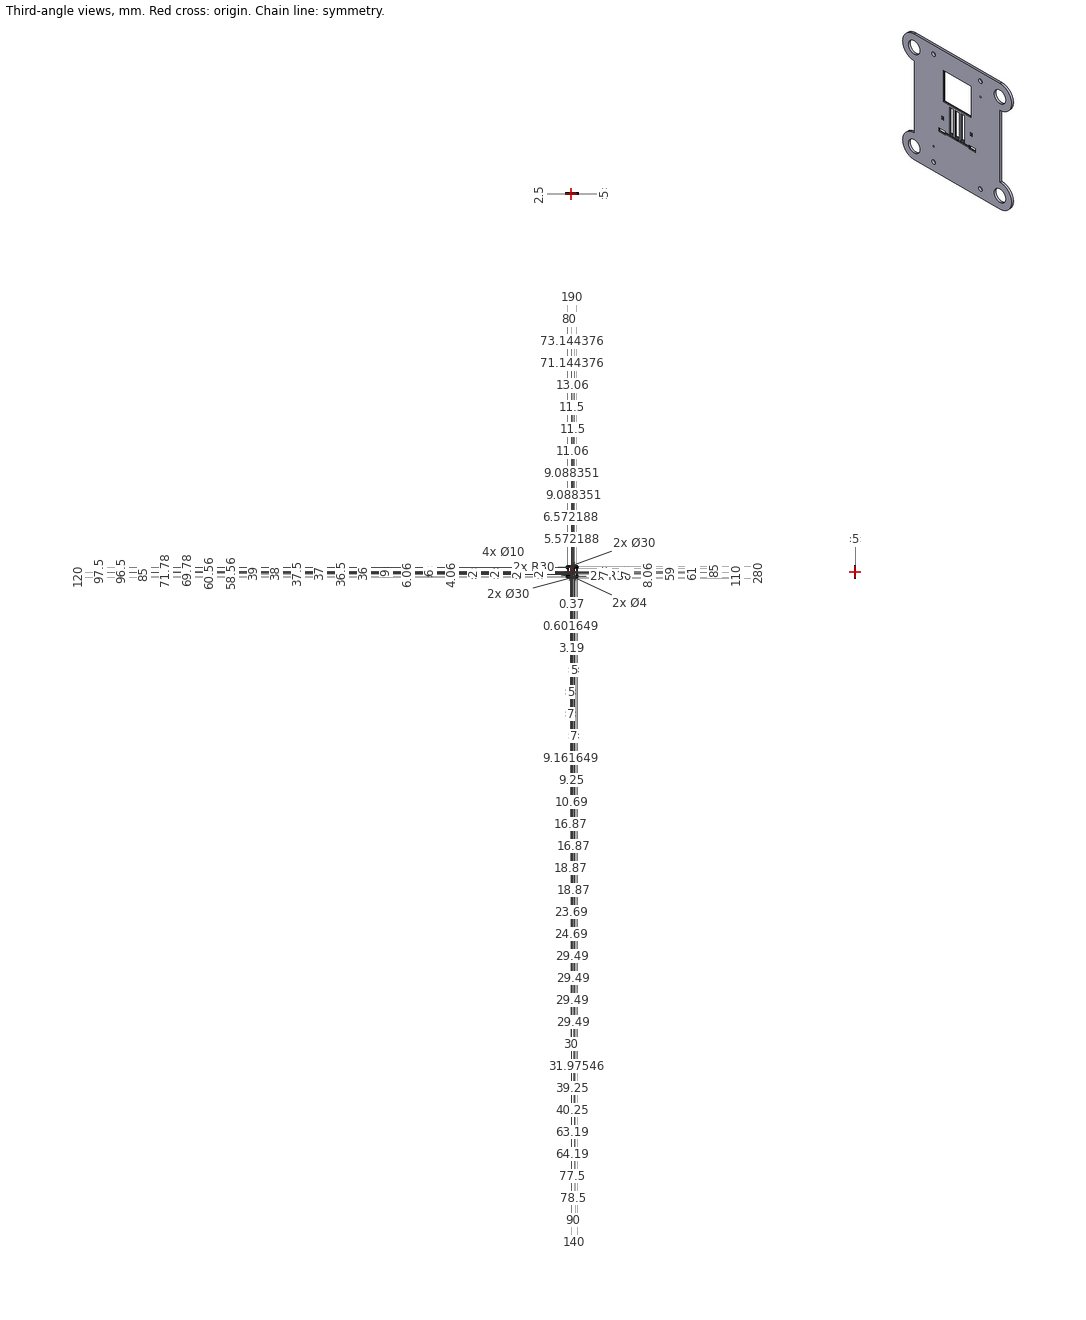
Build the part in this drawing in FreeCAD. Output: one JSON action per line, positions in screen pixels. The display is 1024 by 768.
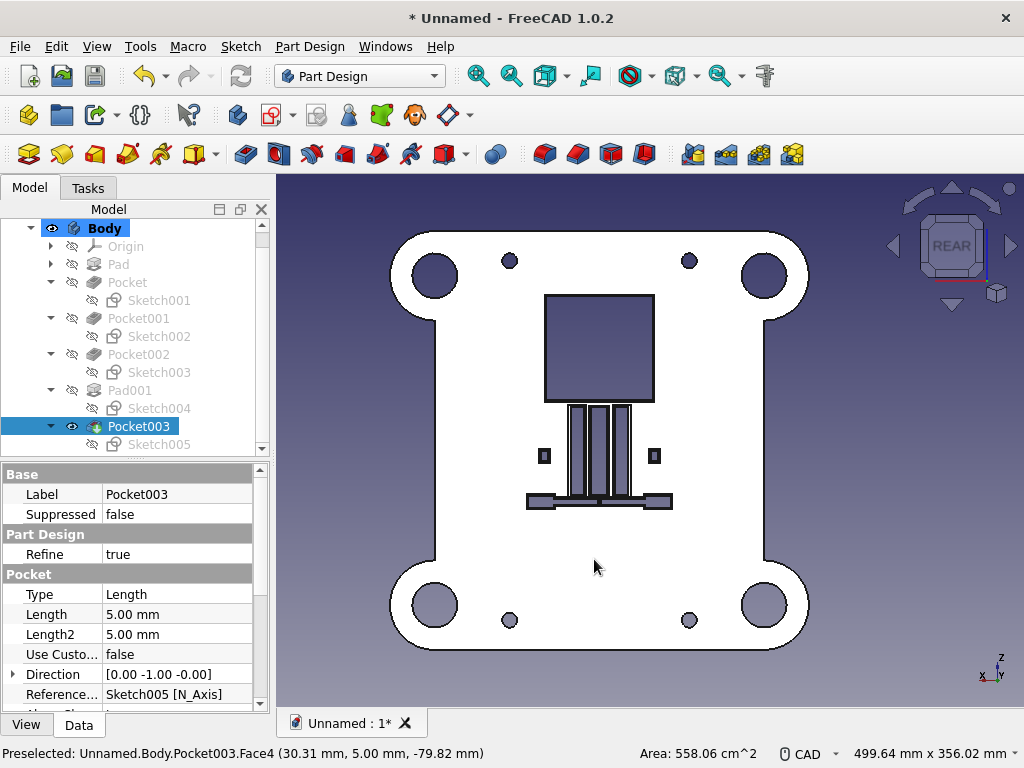
{"action": "left_click", "coordinate": [270, 116]}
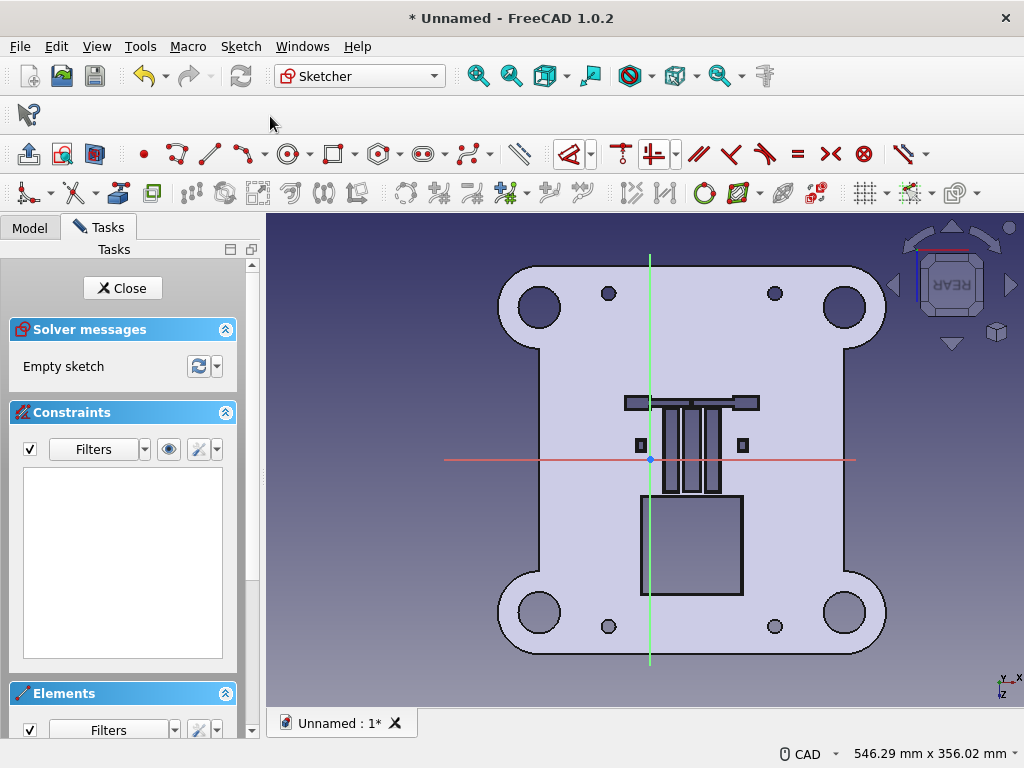
{"action": "left_click", "coordinate": [288, 154]}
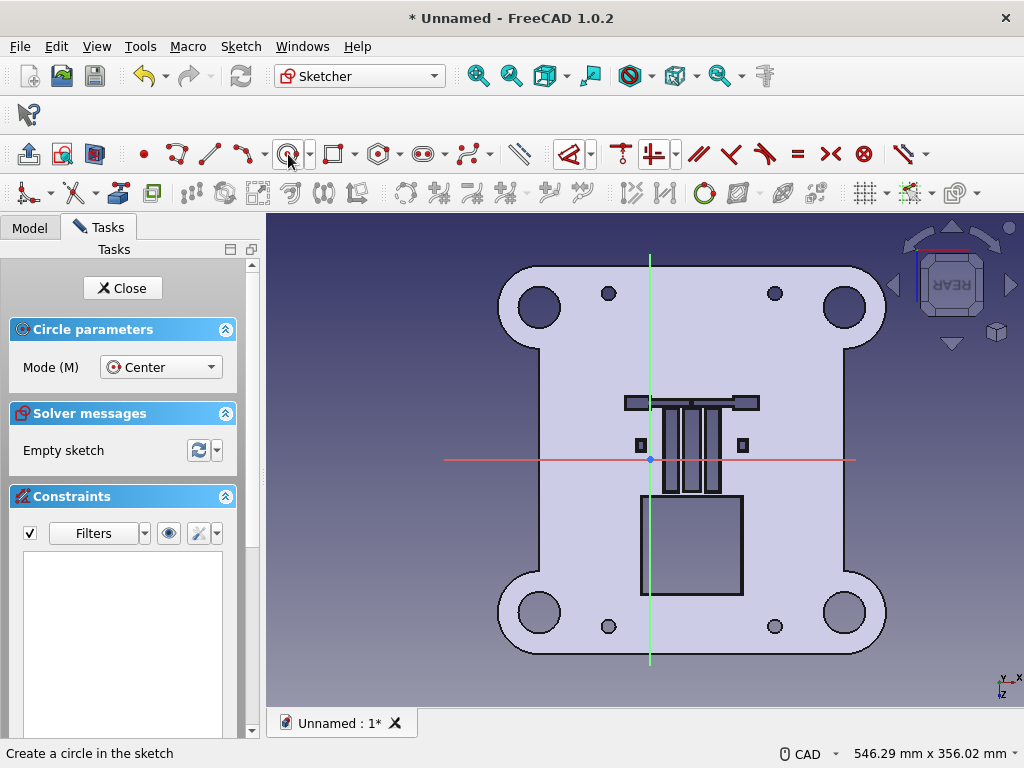
{"action": "scroll", "coordinate": [609, 342], "scroll_direction": "up", "scroll_amount": 11}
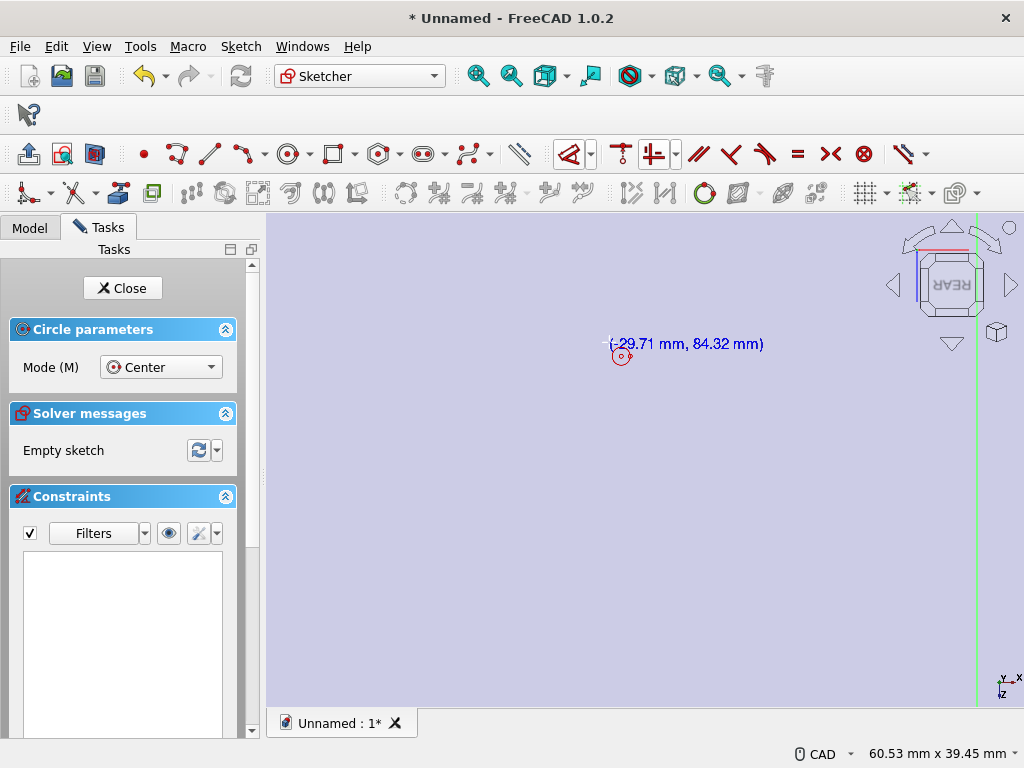
{"action": "scroll", "coordinate": [455, 312], "scroll_direction": "down", "scroll_amount": 10}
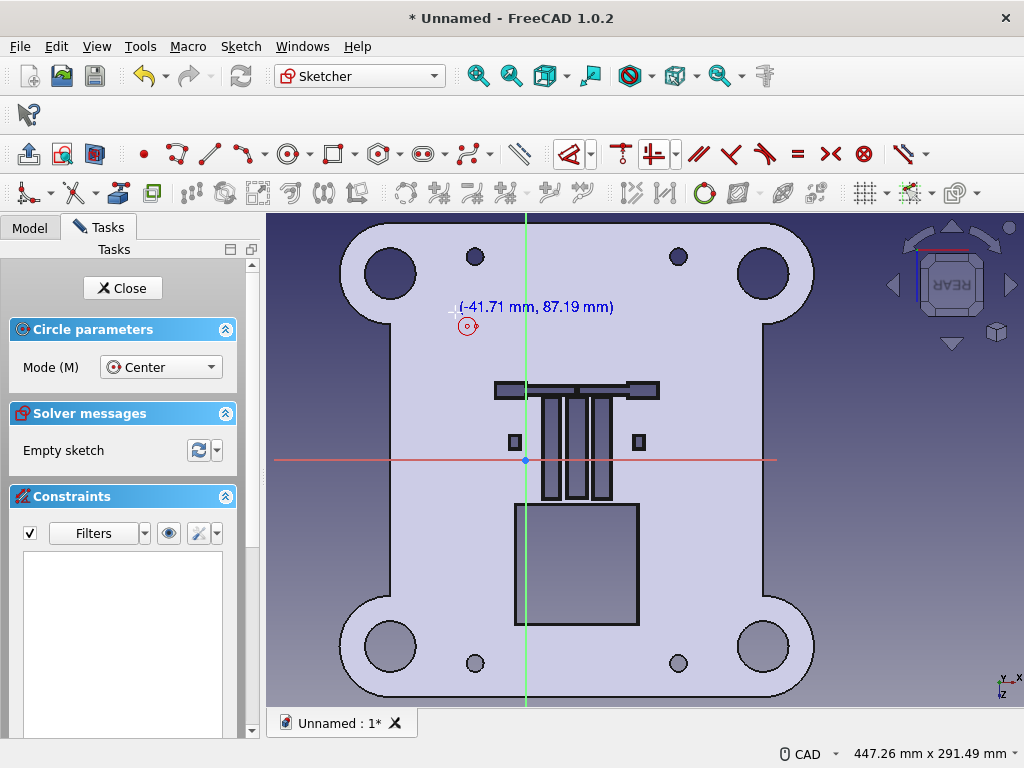
{"action": "left_click", "coordinate": [475, 316]}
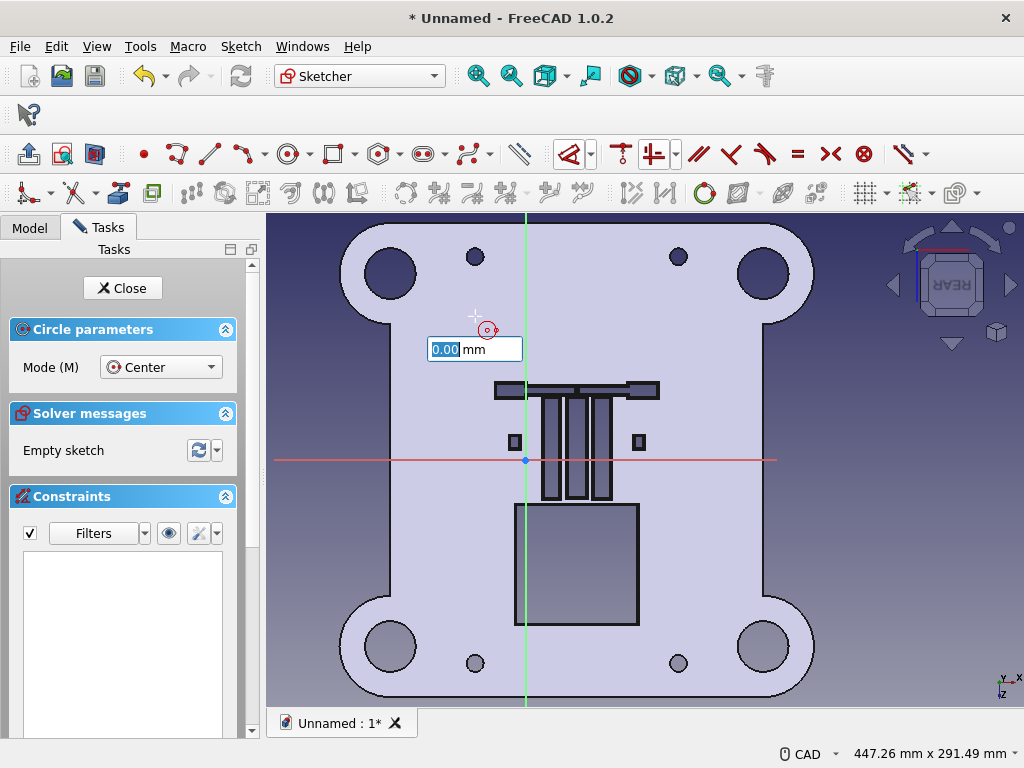
{"action": "scroll", "coordinate": [477, 314], "scroll_direction": "up", "scroll_amount": 8}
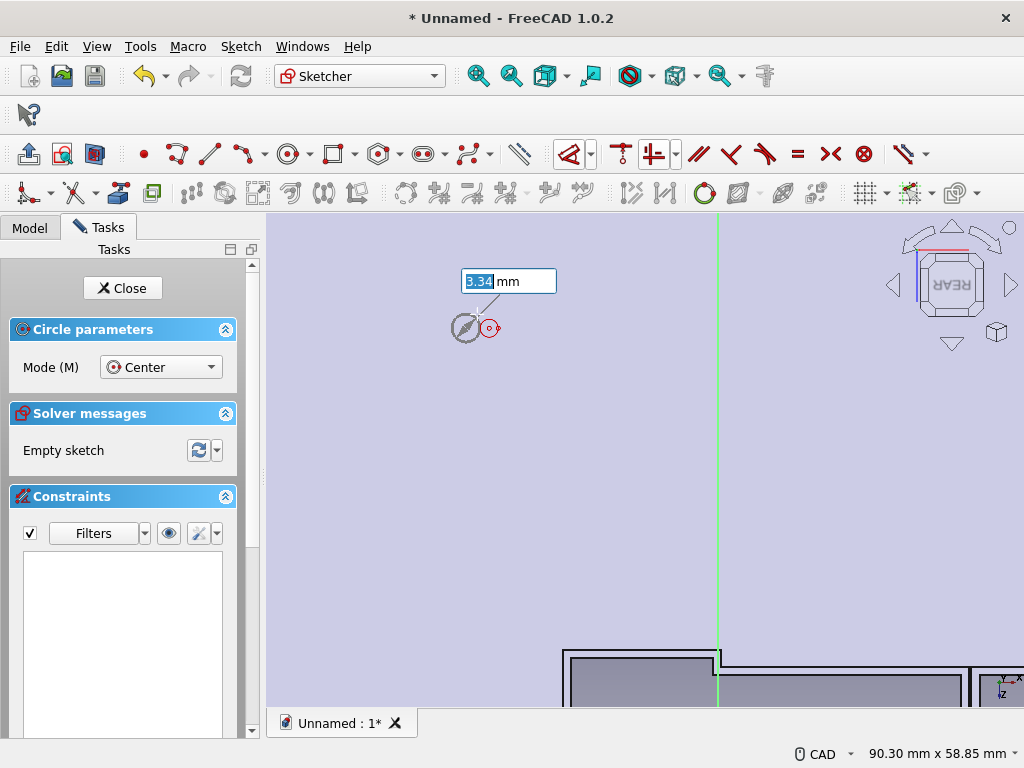
{"action": "left_click", "coordinate": [478, 311]}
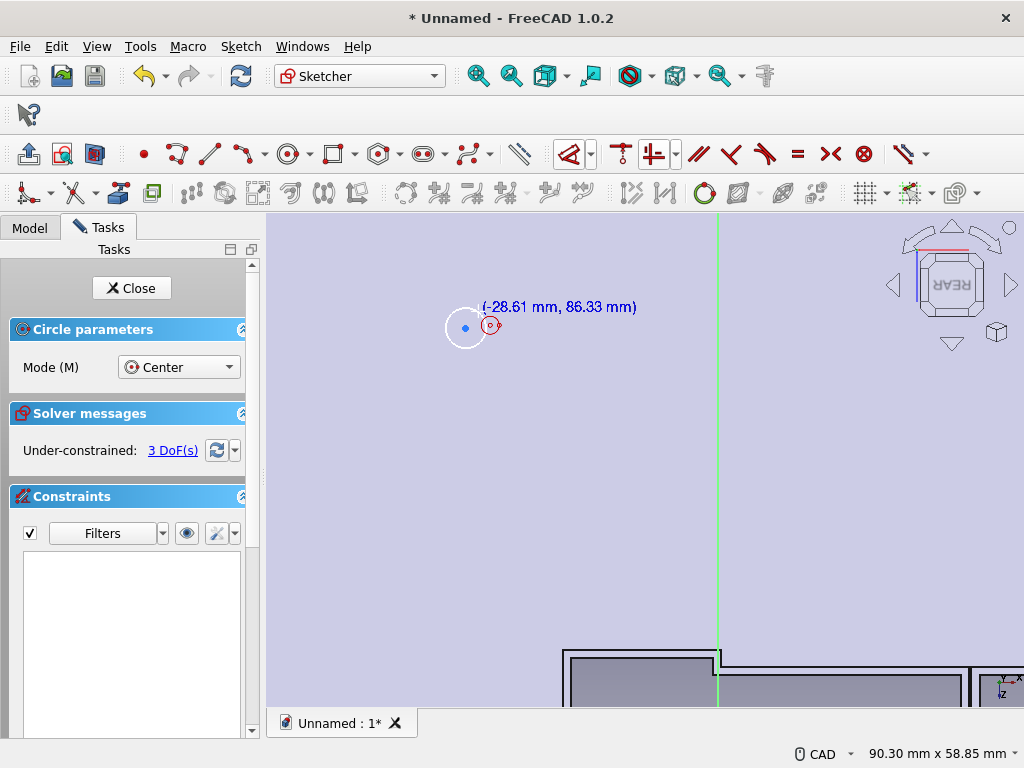
{"action": "scroll", "coordinate": [477, 314], "scroll_direction": "down", "scroll_amount": 8}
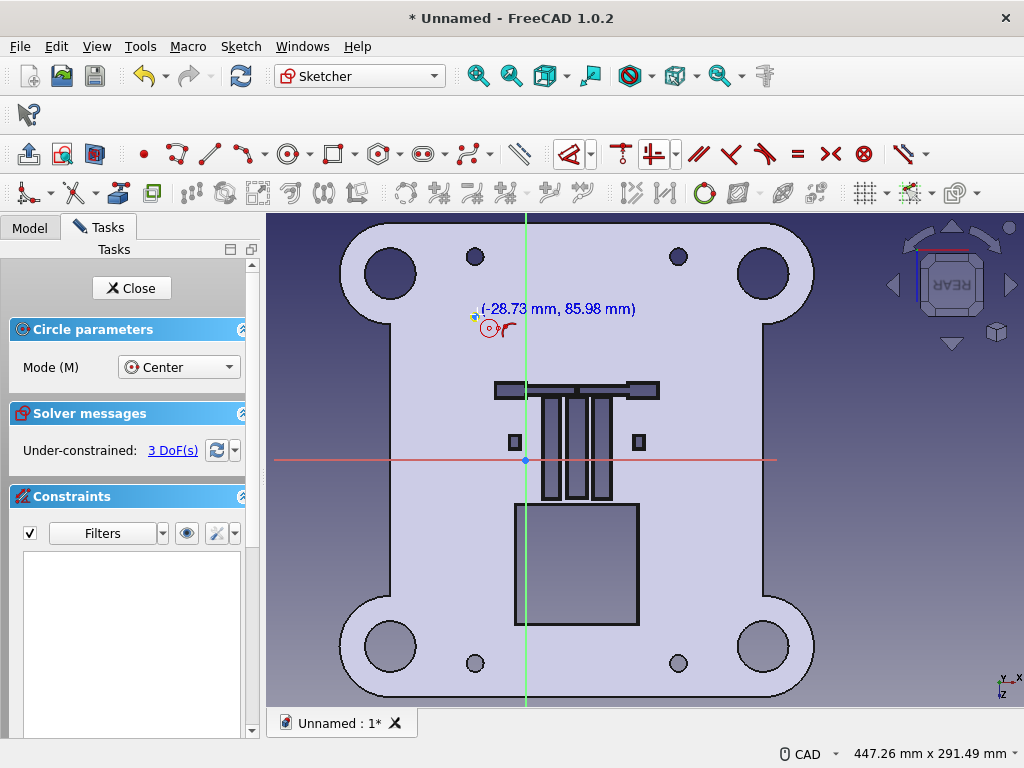
{"action": "scroll", "coordinate": [678, 604], "scroll_direction": "up", "scroll_amount": 10}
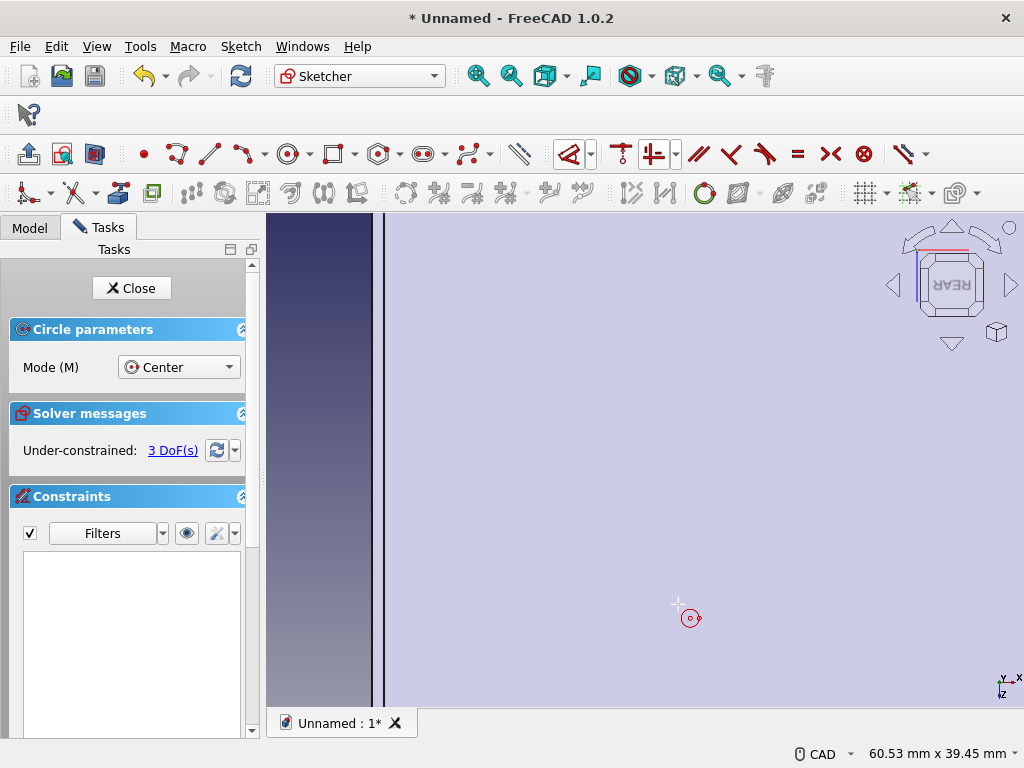
{"action": "scroll", "coordinate": [678, 605], "scroll_direction": "down", "scroll_amount": 10}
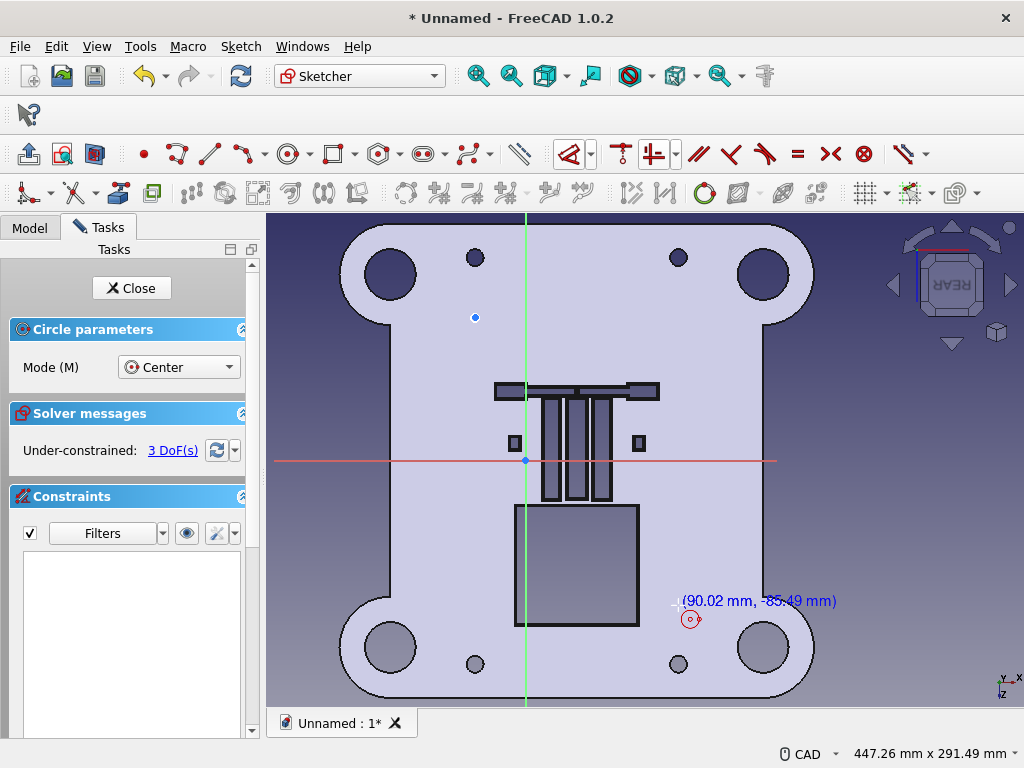
{"action": "left_click", "coordinate": [678, 605]}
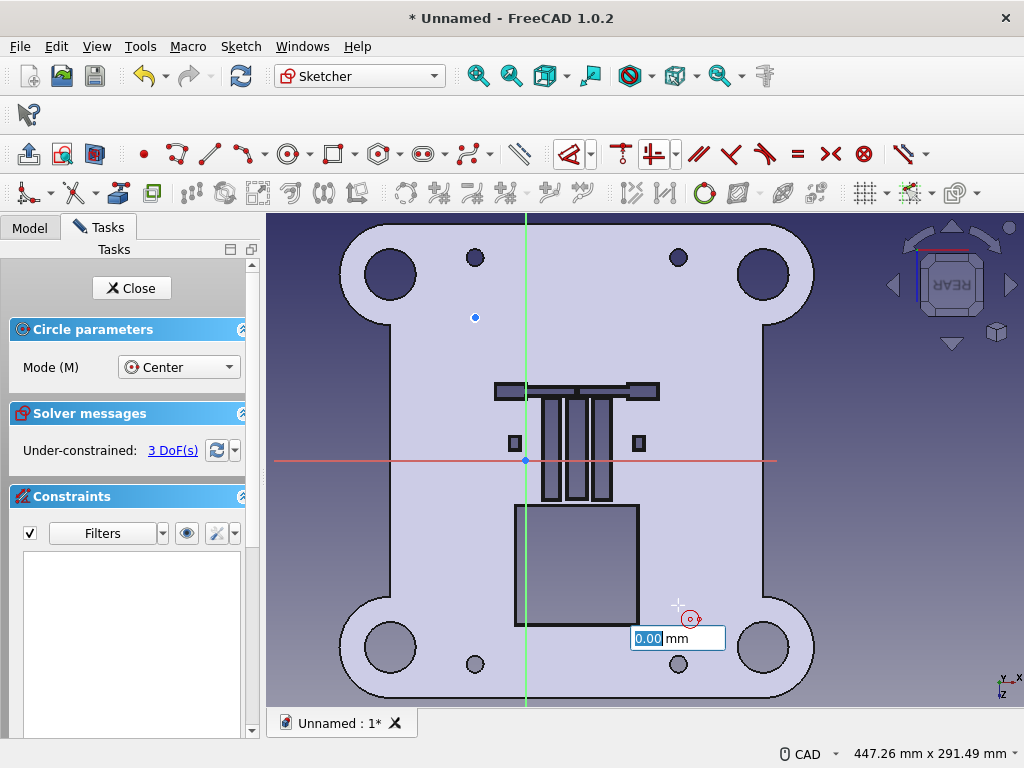
{"action": "scroll", "coordinate": [681, 603], "scroll_direction": "up", "scroll_amount": 8}